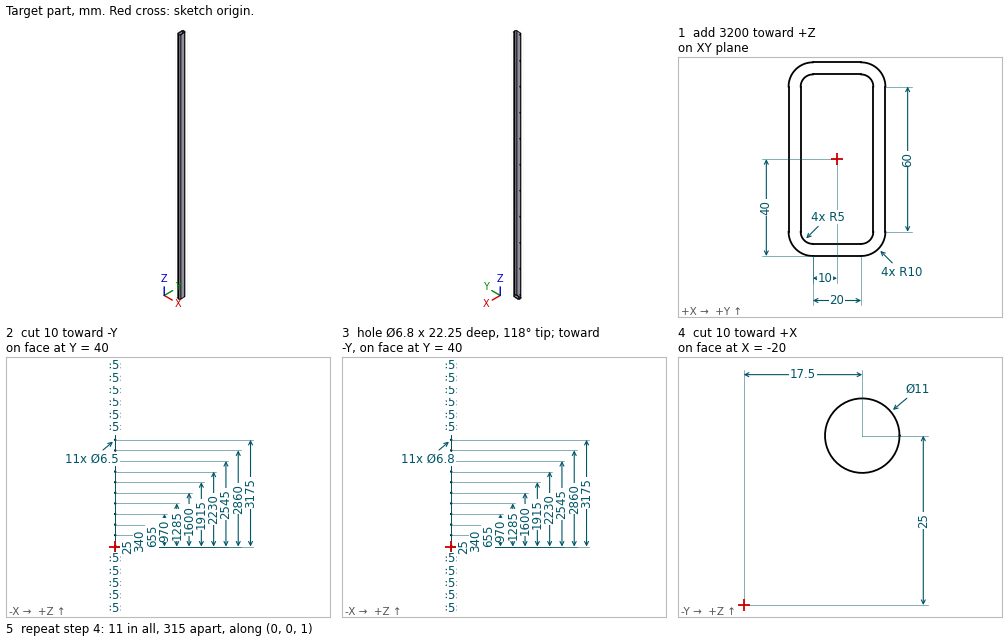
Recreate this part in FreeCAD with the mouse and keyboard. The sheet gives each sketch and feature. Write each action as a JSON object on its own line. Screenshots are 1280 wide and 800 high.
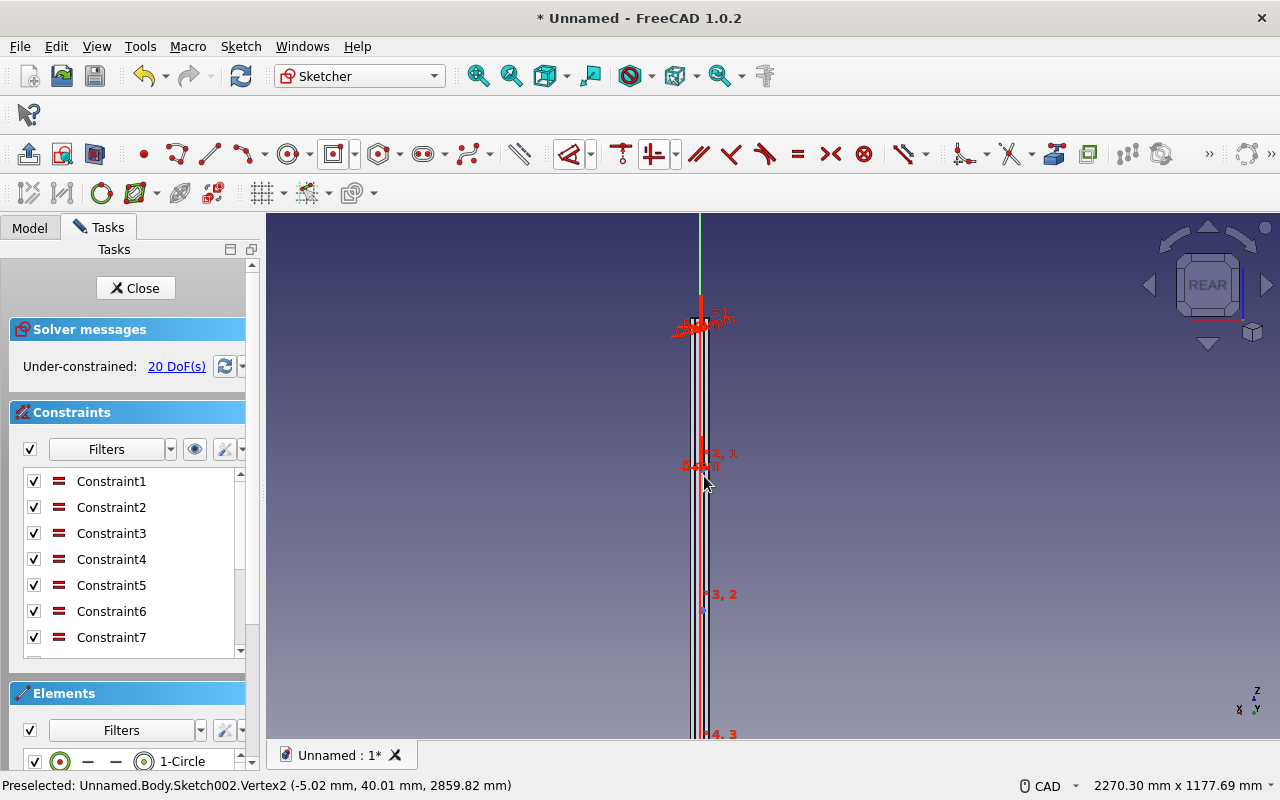
{"action": "scroll", "coordinate": [705, 292], "scroll_direction": "down", "scroll_amount": 7}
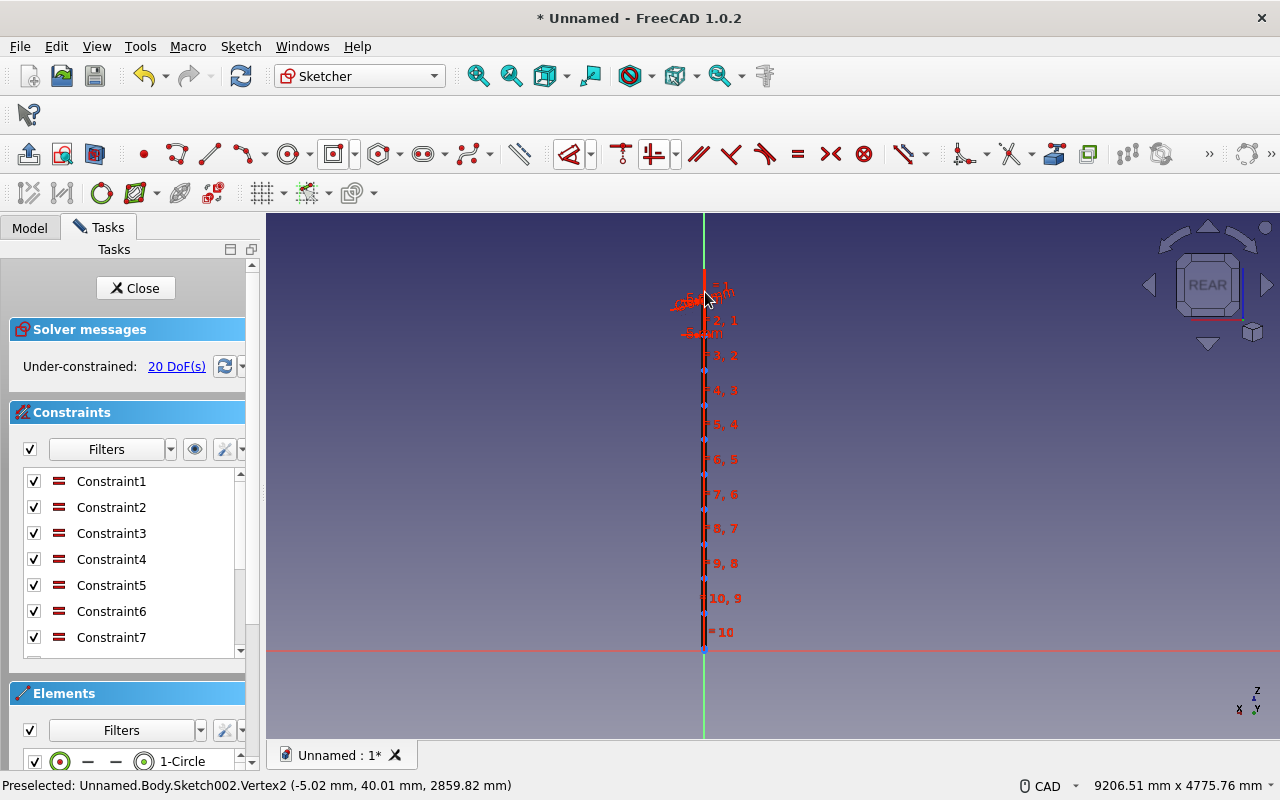
{"action": "scroll", "coordinate": [705, 371], "scroll_direction": "up", "scroll_amount": 22}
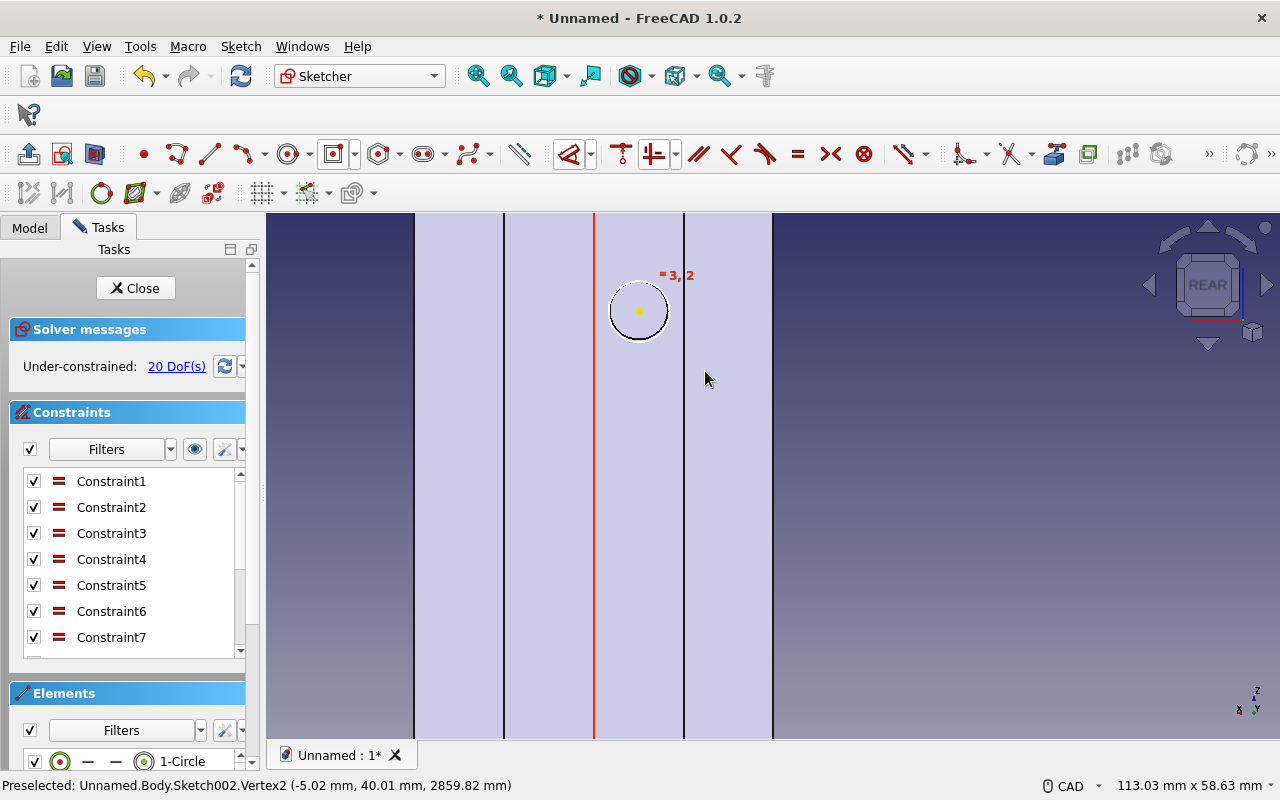
{"action": "left_click", "coordinate": [639, 312]}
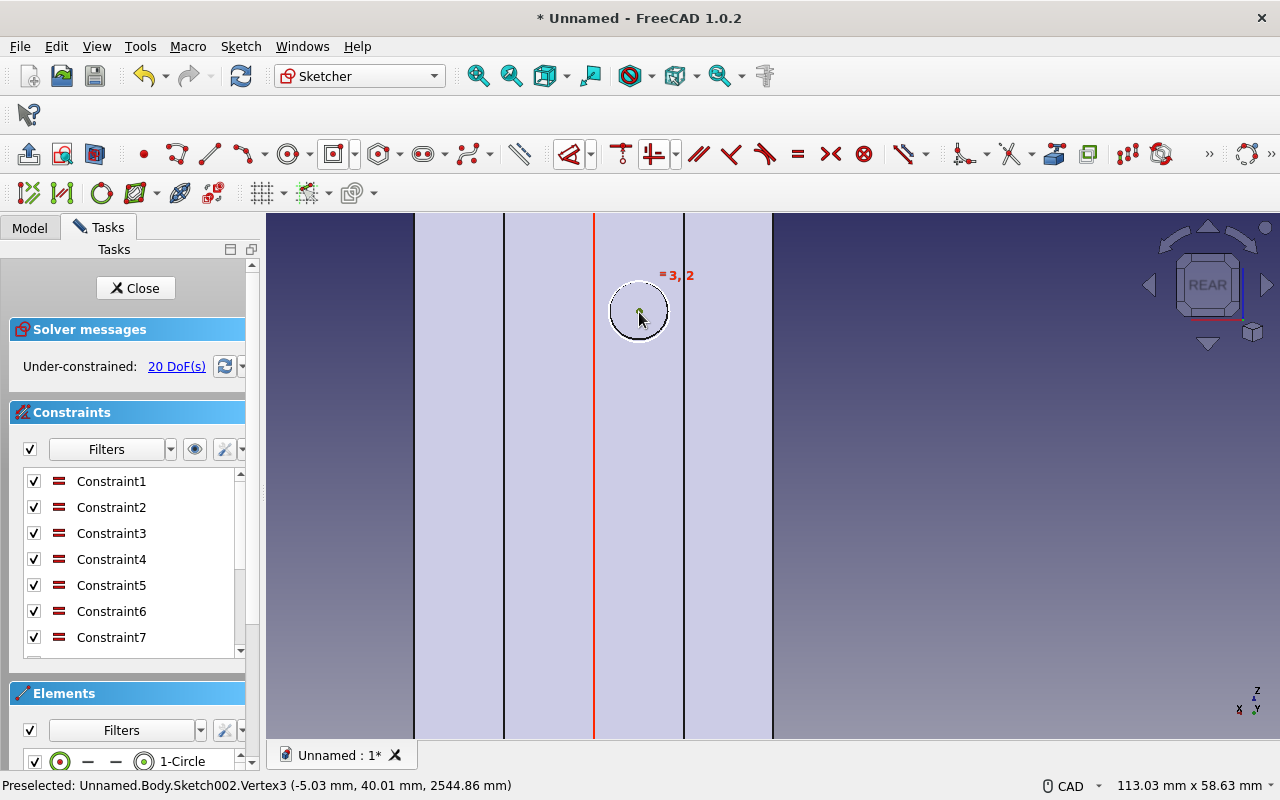
{"action": "left_click", "coordinate": [590, 154]}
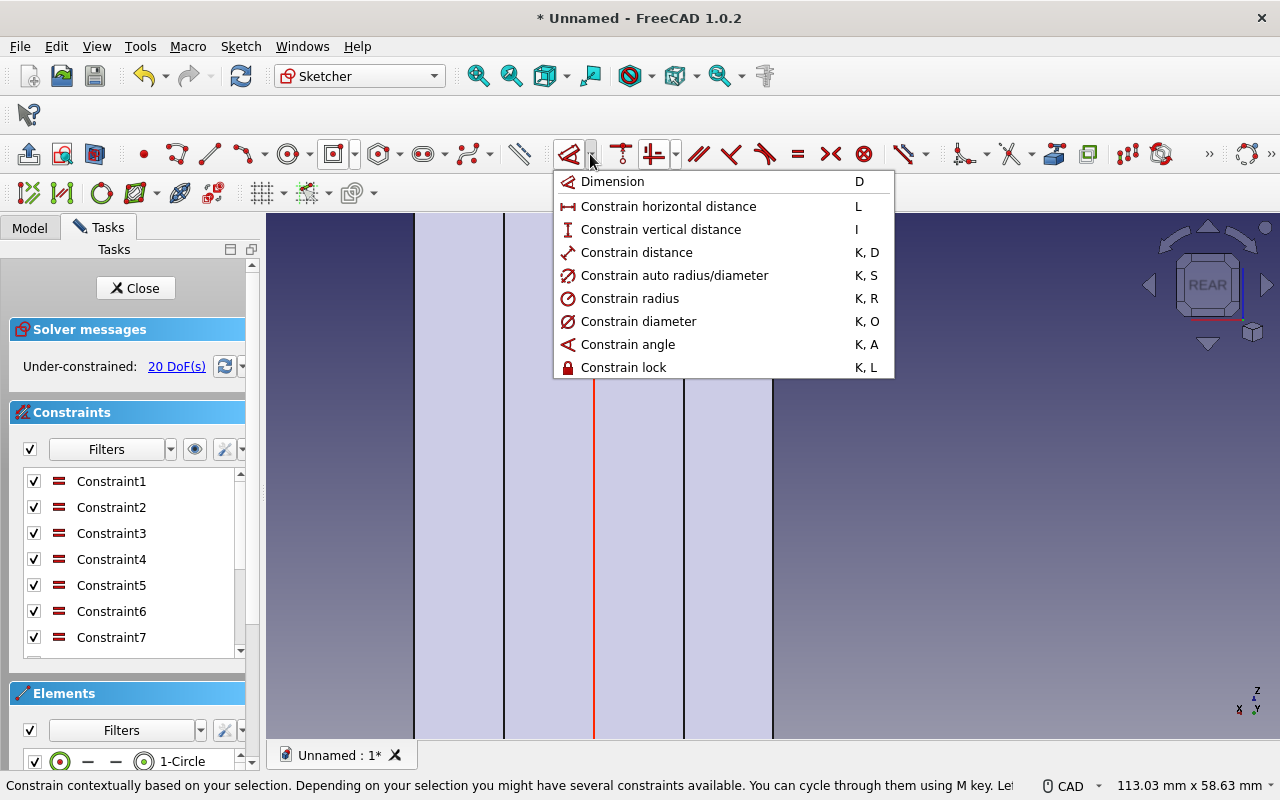
{"action": "left_click", "coordinate": [724, 206]}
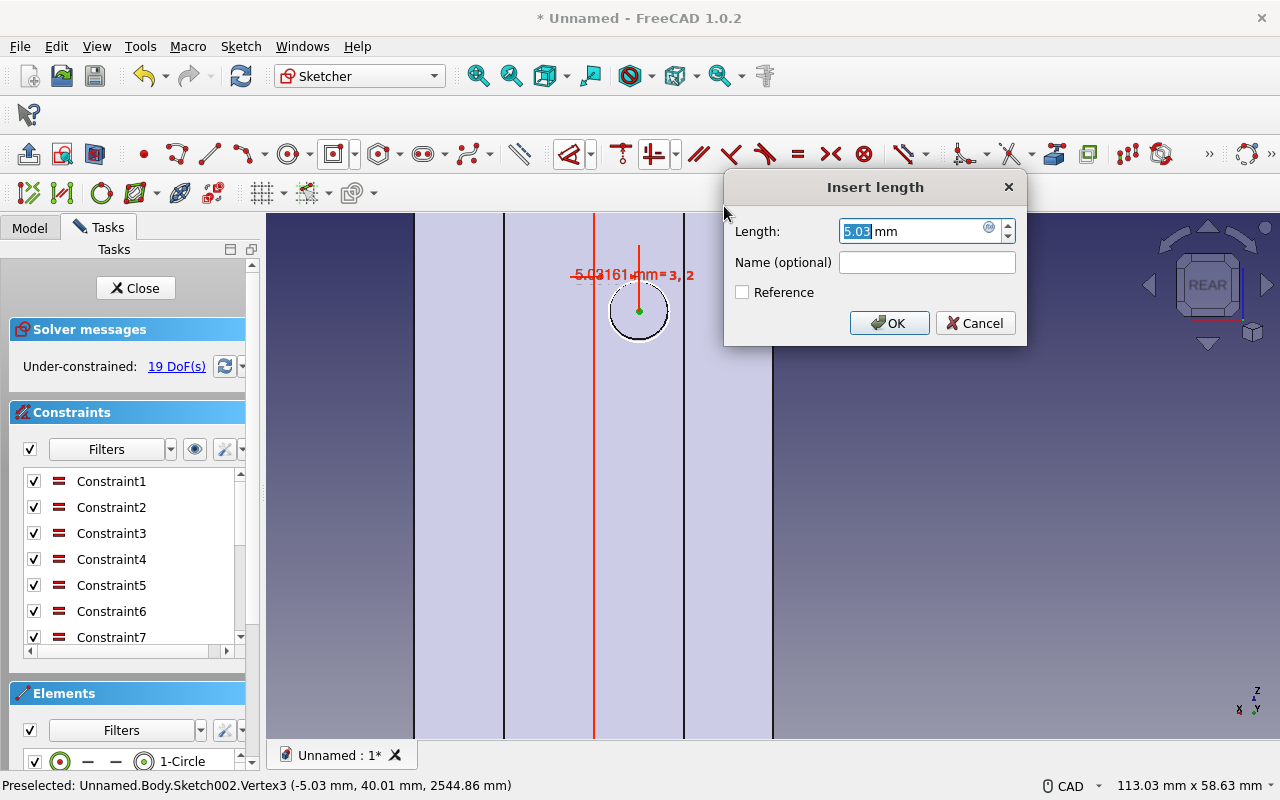
{"action": "type", "text": "5"}
{"action": "key", "text": "Return"}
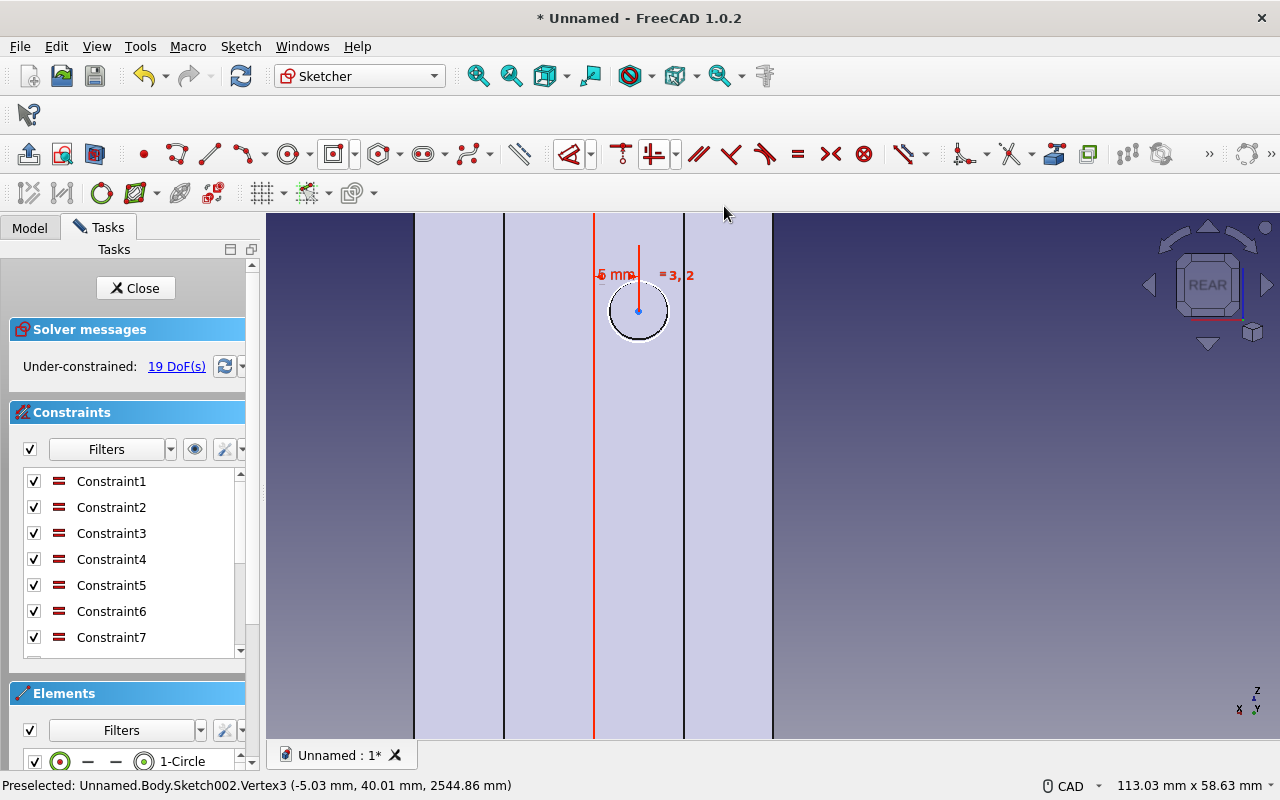
{"action": "scroll", "coordinate": [704, 476], "scroll_direction": "down", "scroll_amount": 15}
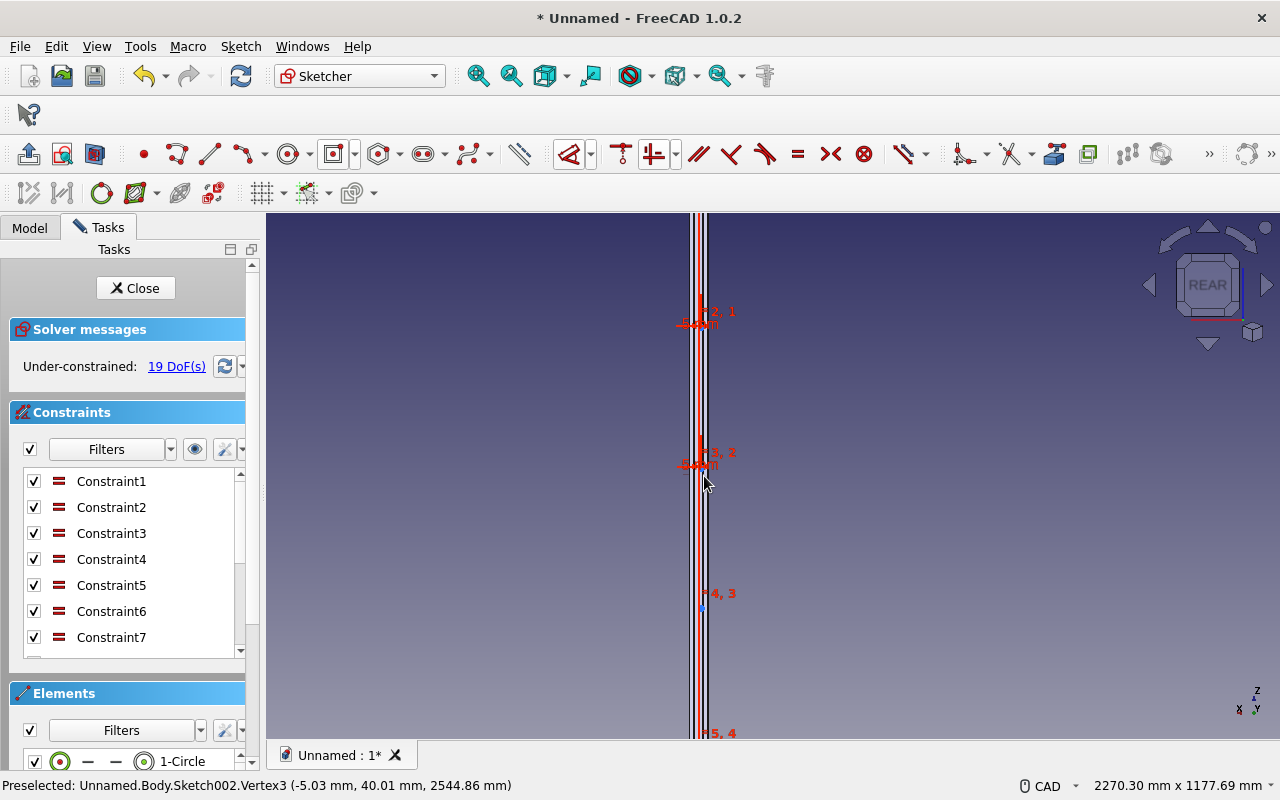
{"action": "scroll", "coordinate": [706, 339], "scroll_direction": "down", "scroll_amount": 7}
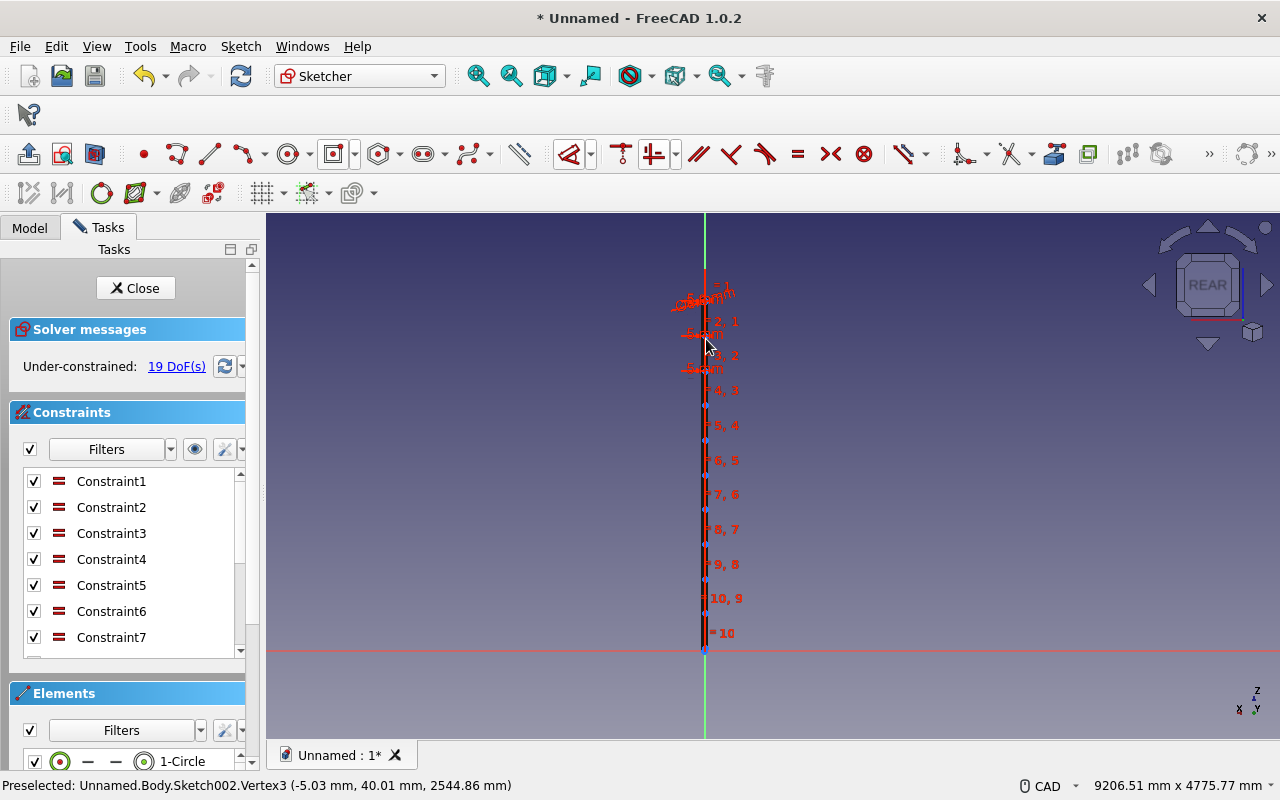
{"action": "scroll", "coordinate": [705, 406], "scroll_direction": "up", "scroll_amount": 22}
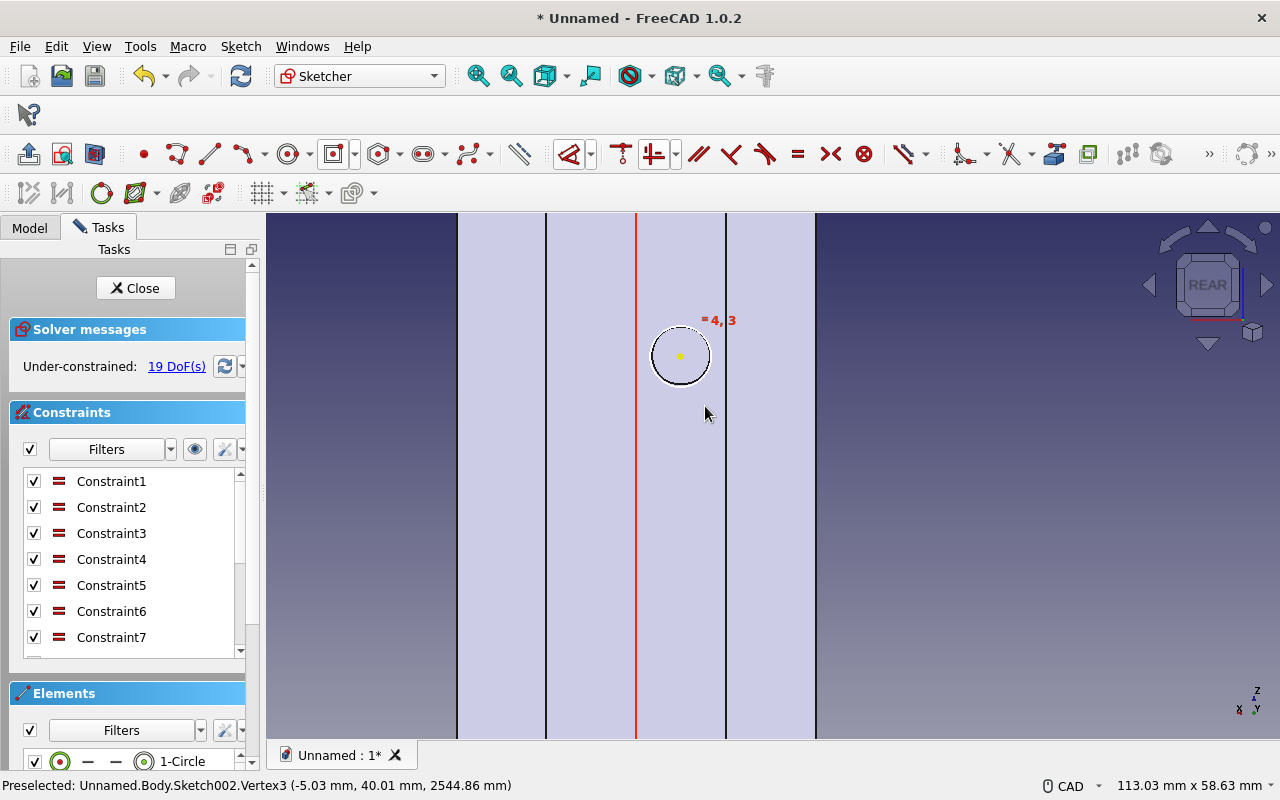
{"action": "left_click", "coordinate": [681, 357]}